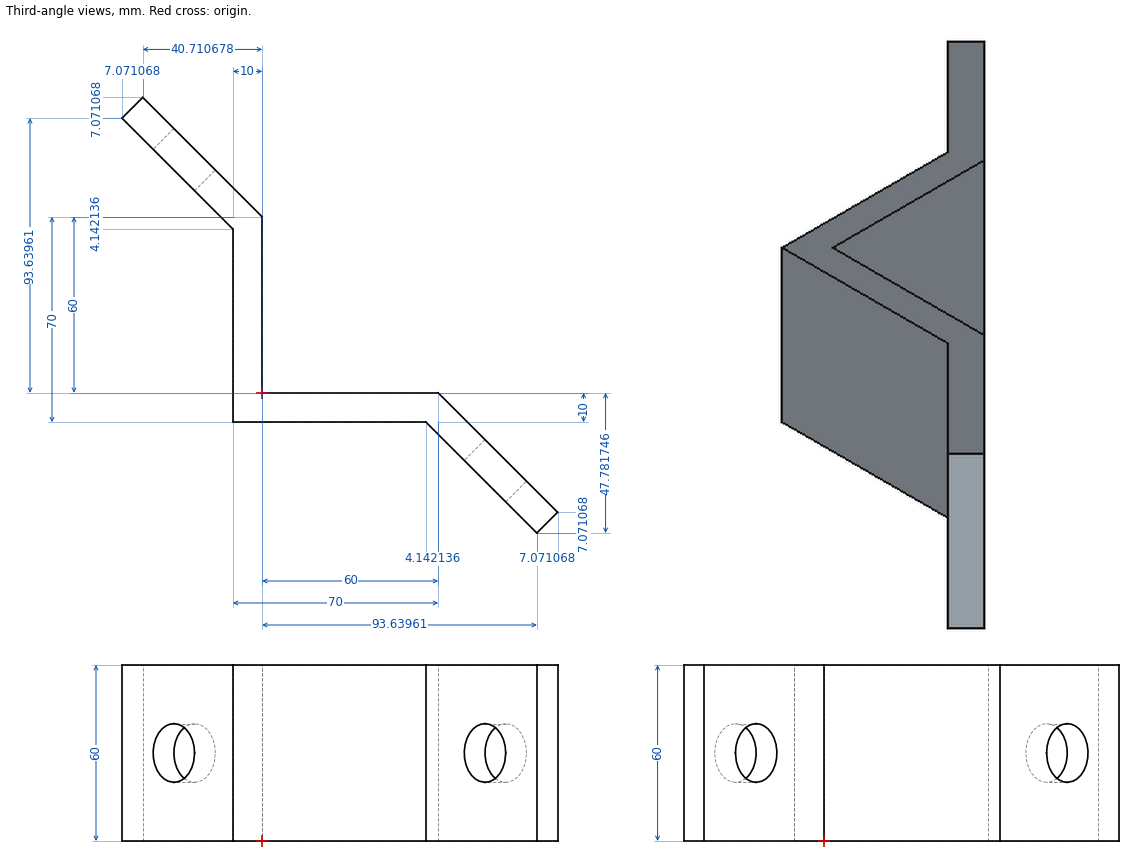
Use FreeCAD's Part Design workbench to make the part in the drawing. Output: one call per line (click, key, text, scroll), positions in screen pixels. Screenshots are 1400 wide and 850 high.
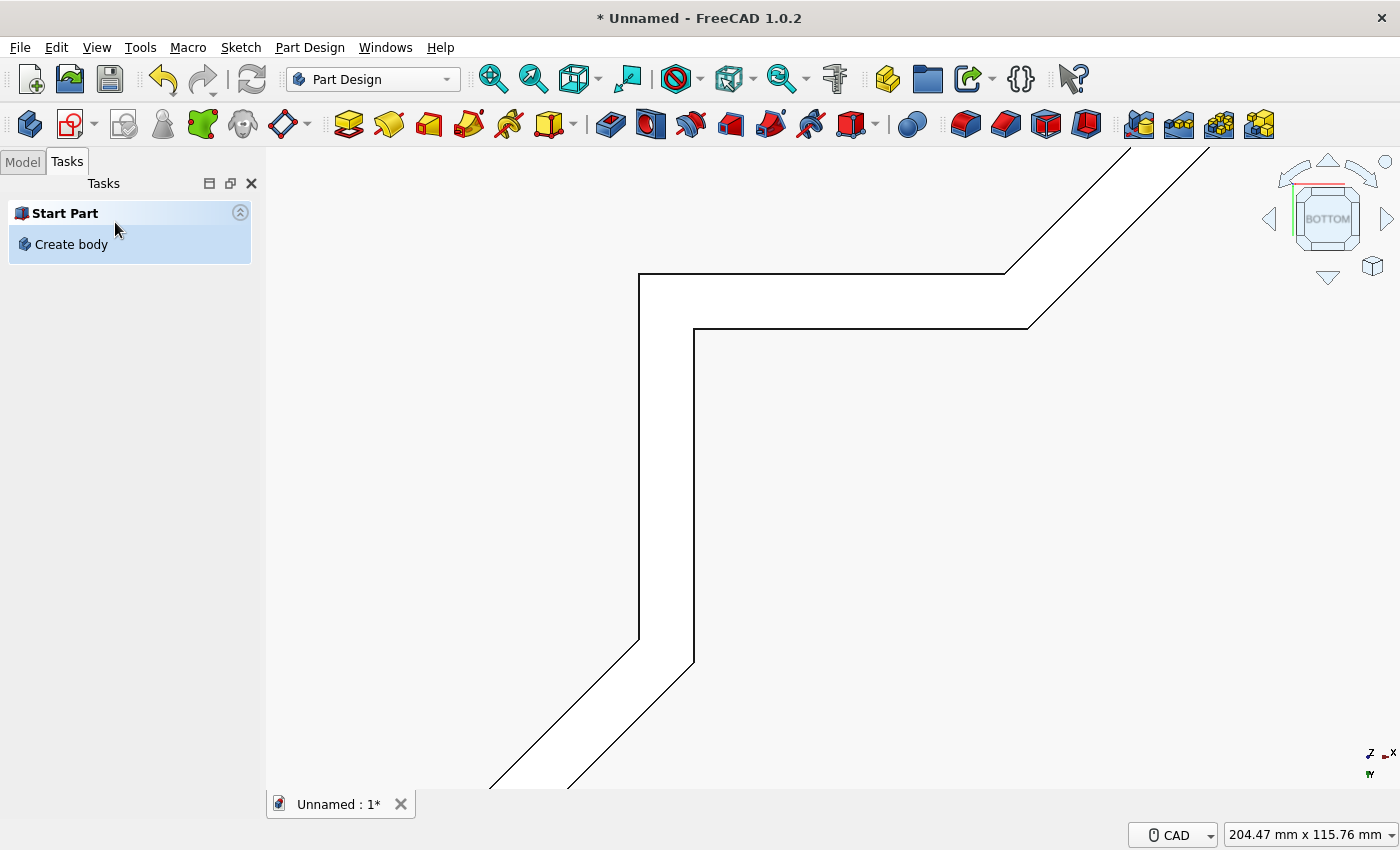
click(494, 80)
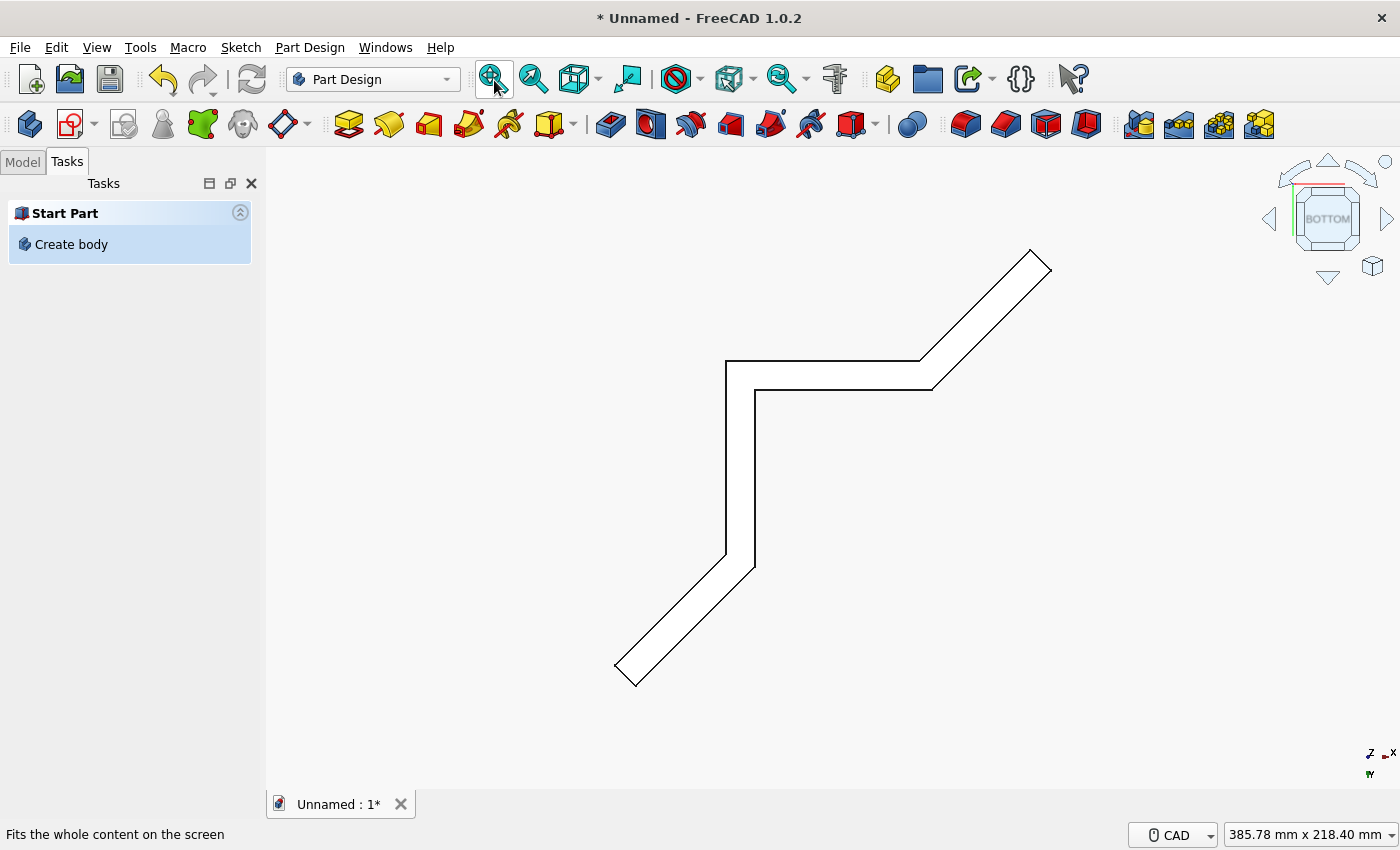
key(6)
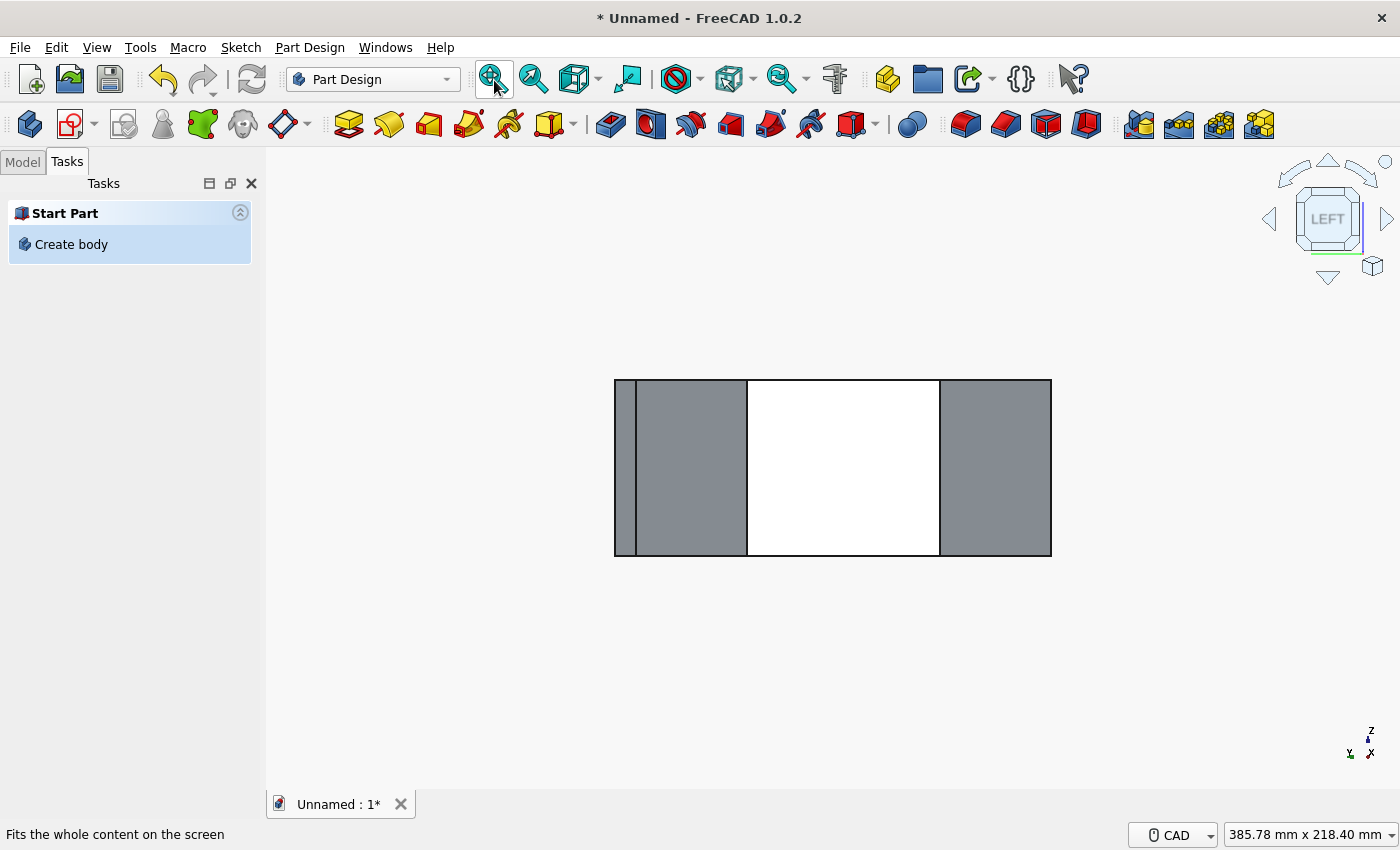
click(494, 80)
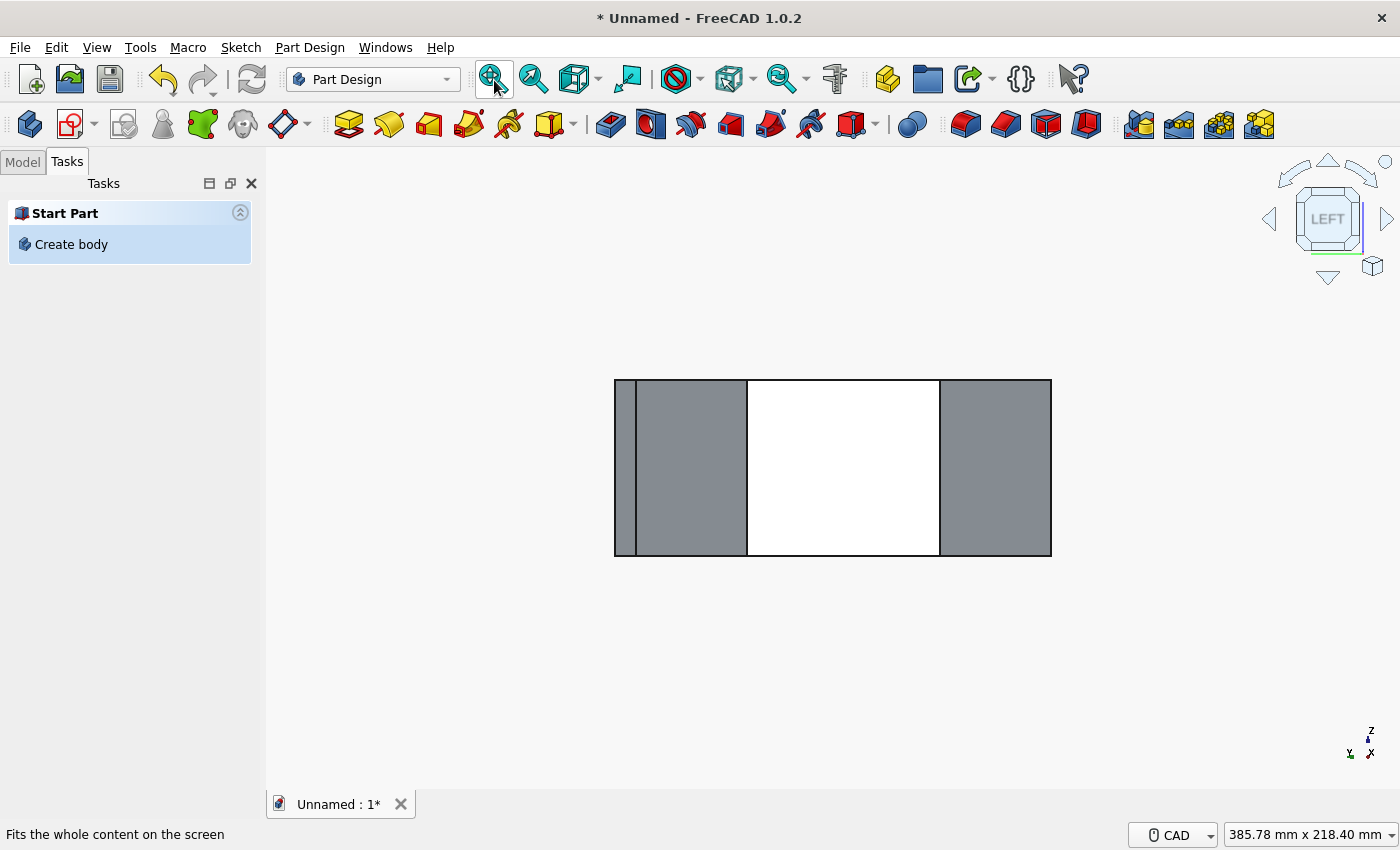
click(691, 467)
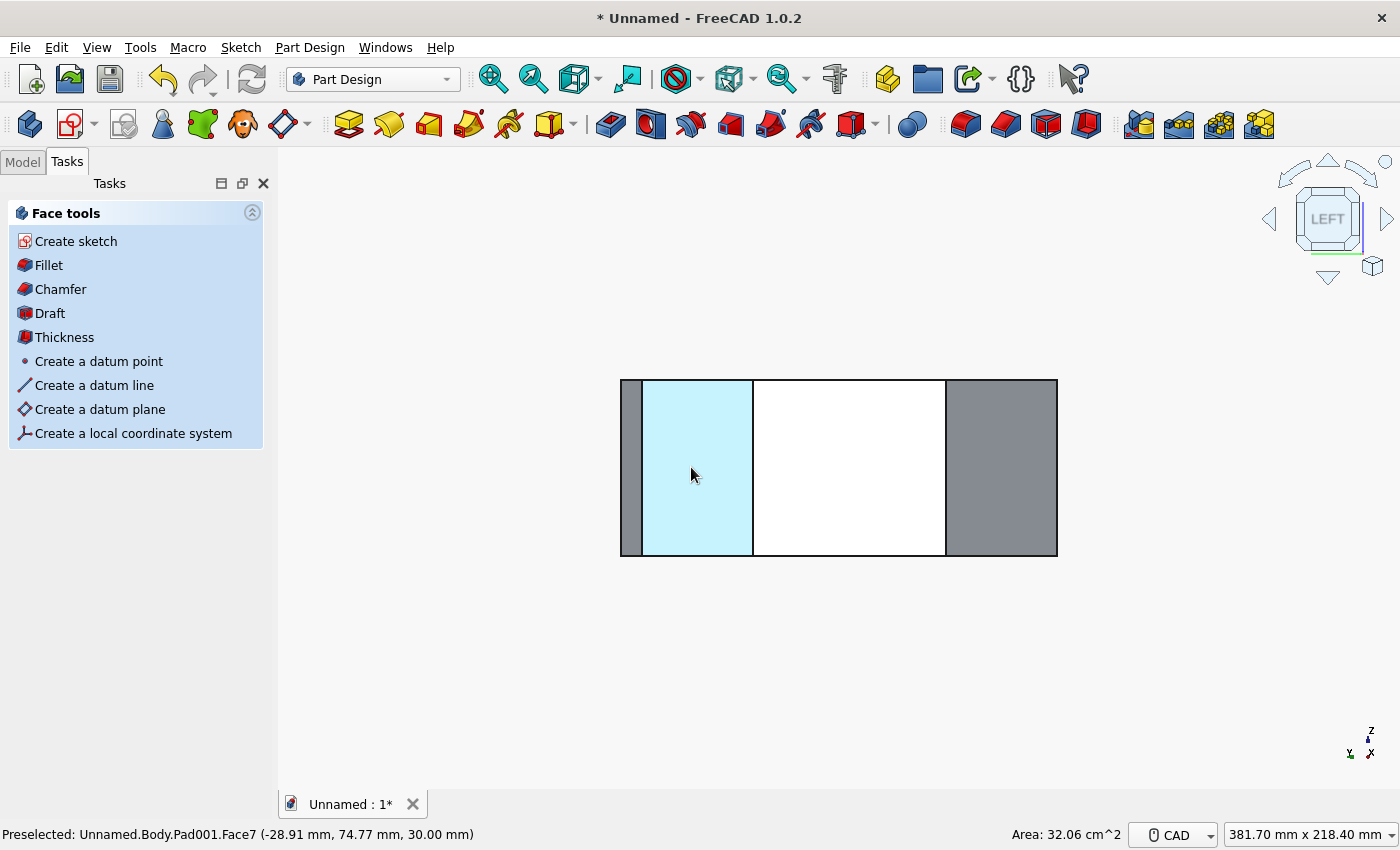
click(70, 124)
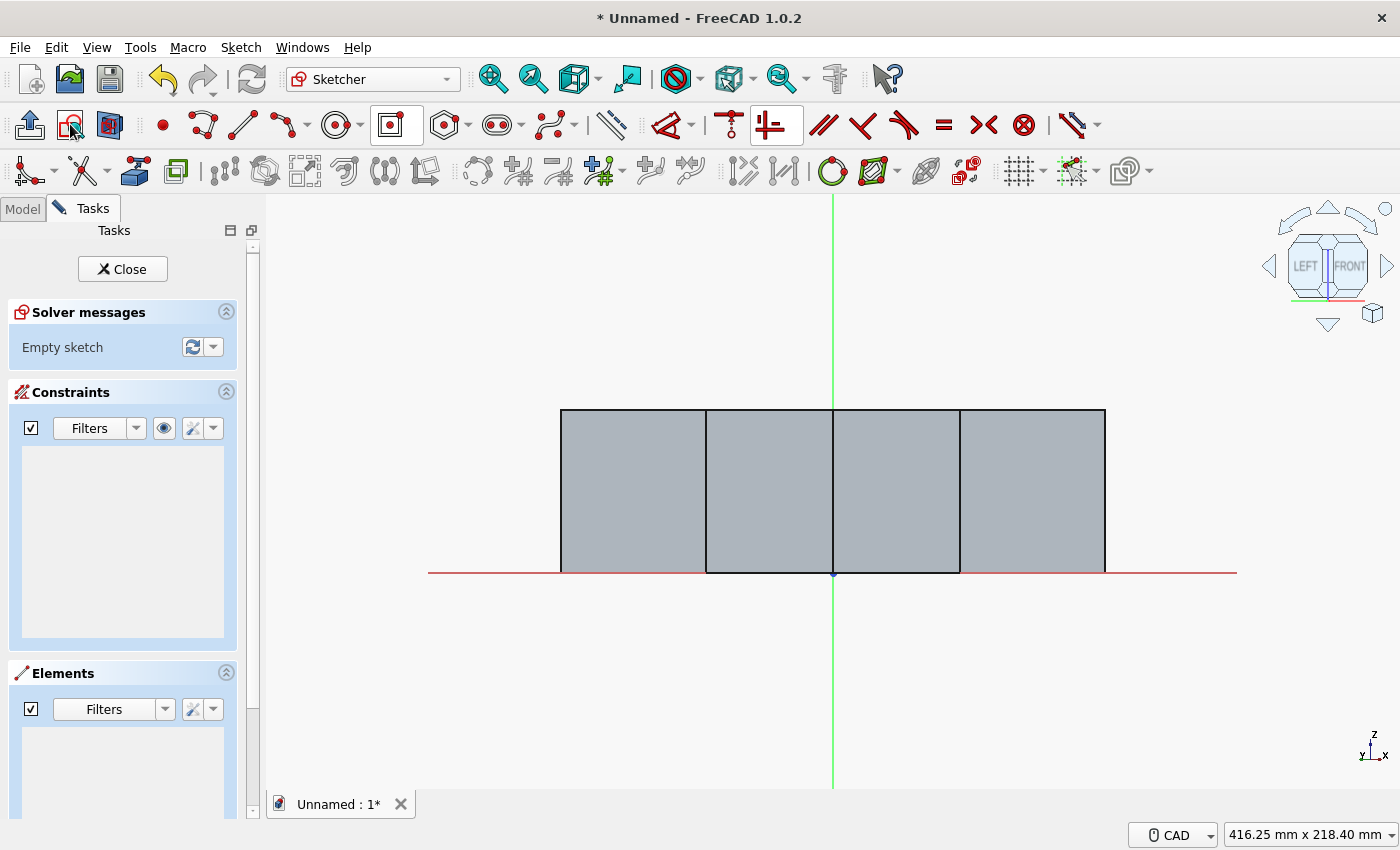
scroll(972, 574, up, 2)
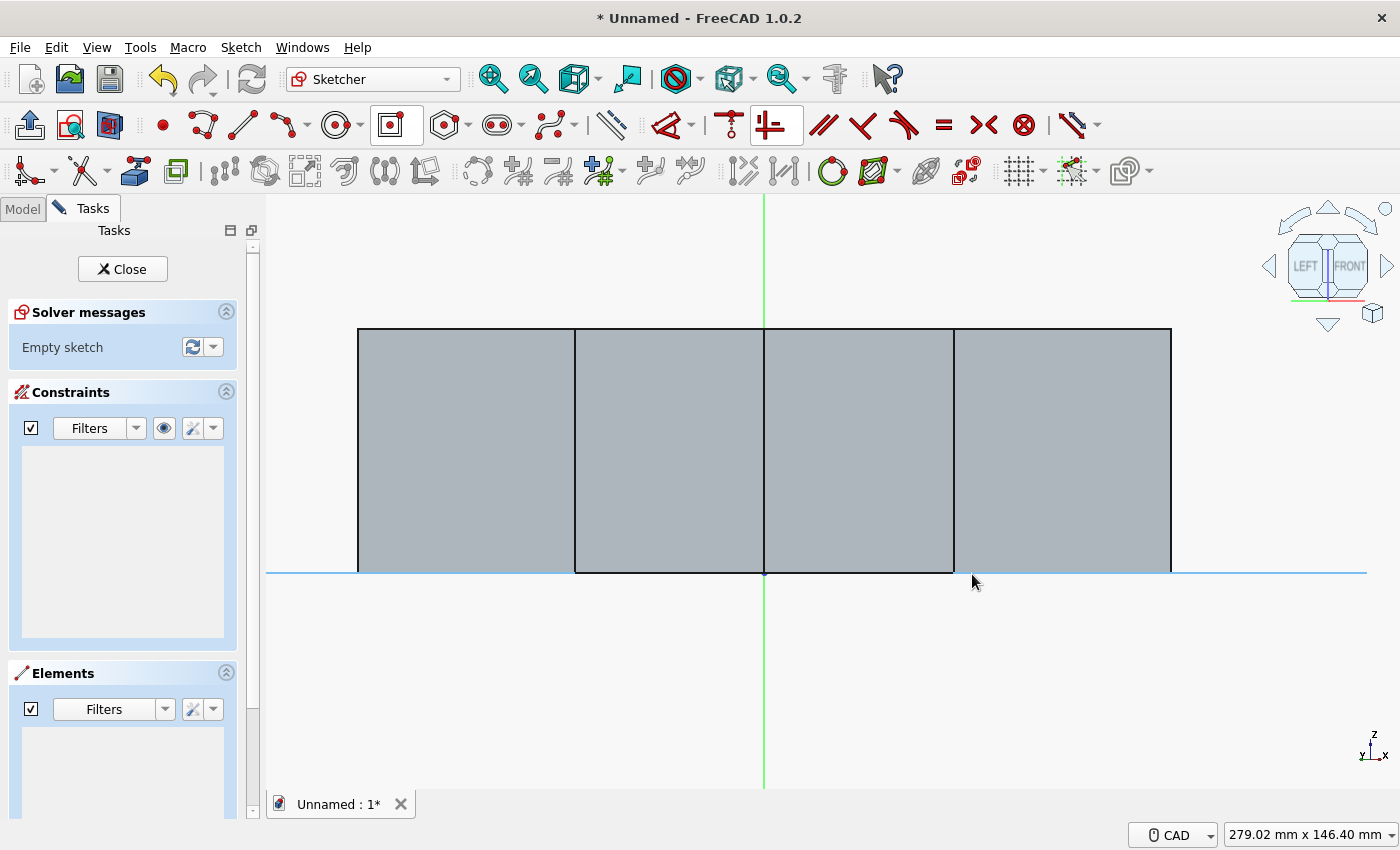
key(g)
key(c)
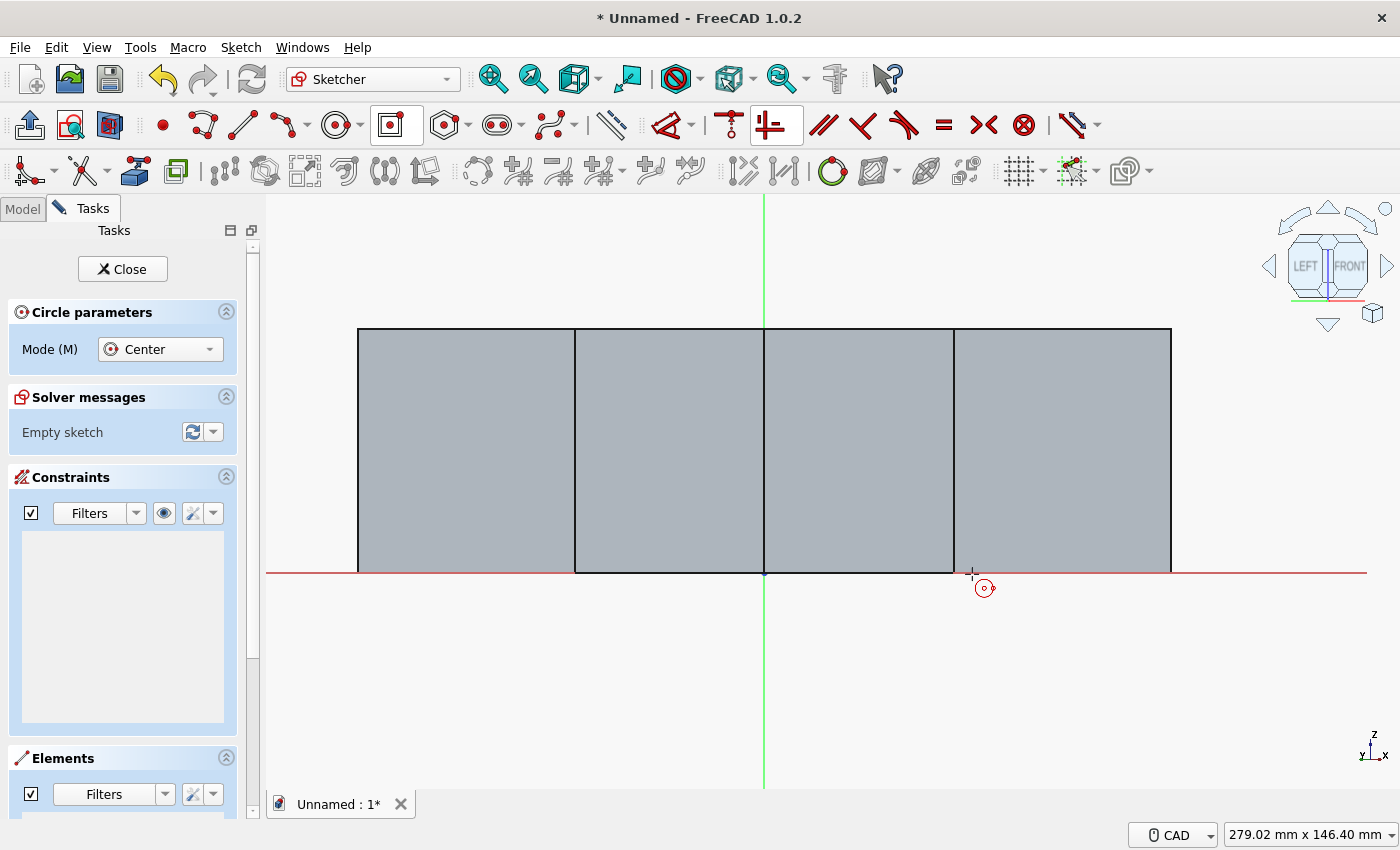
click(460, 451)
click(488, 422)